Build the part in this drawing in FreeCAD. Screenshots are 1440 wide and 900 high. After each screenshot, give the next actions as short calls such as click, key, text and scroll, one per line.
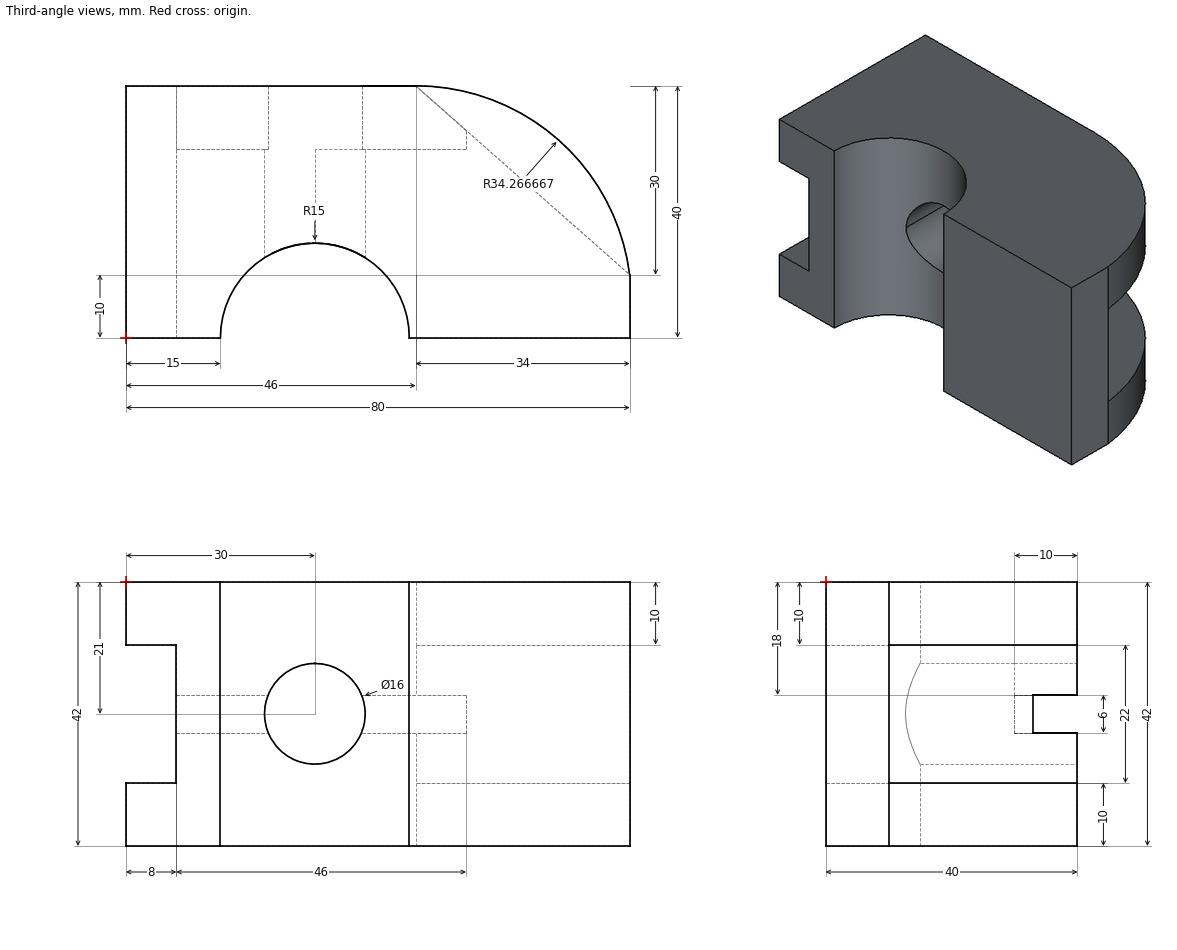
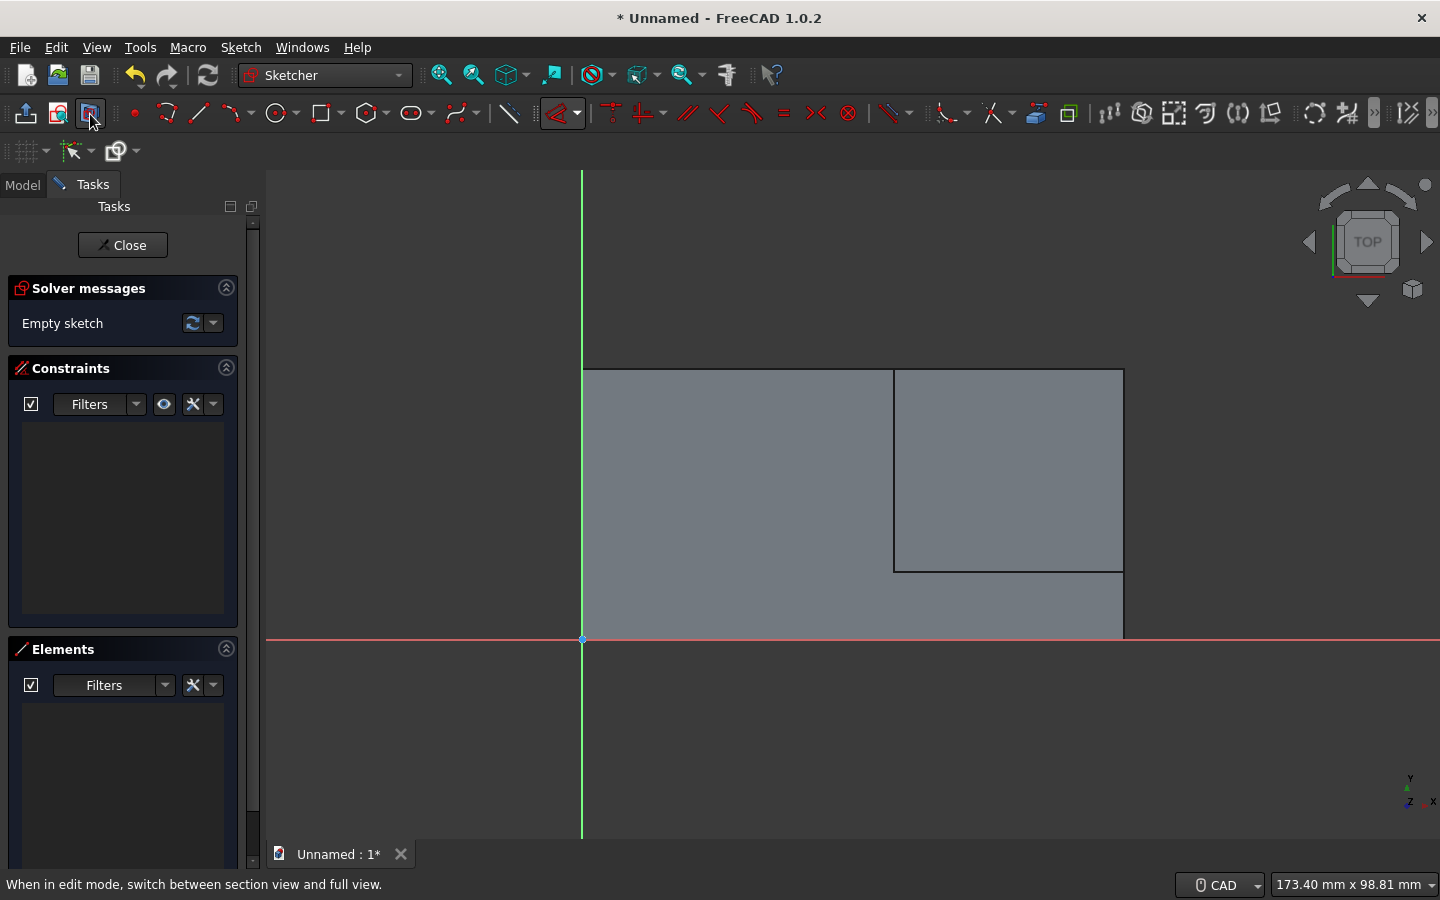
click(168, 114)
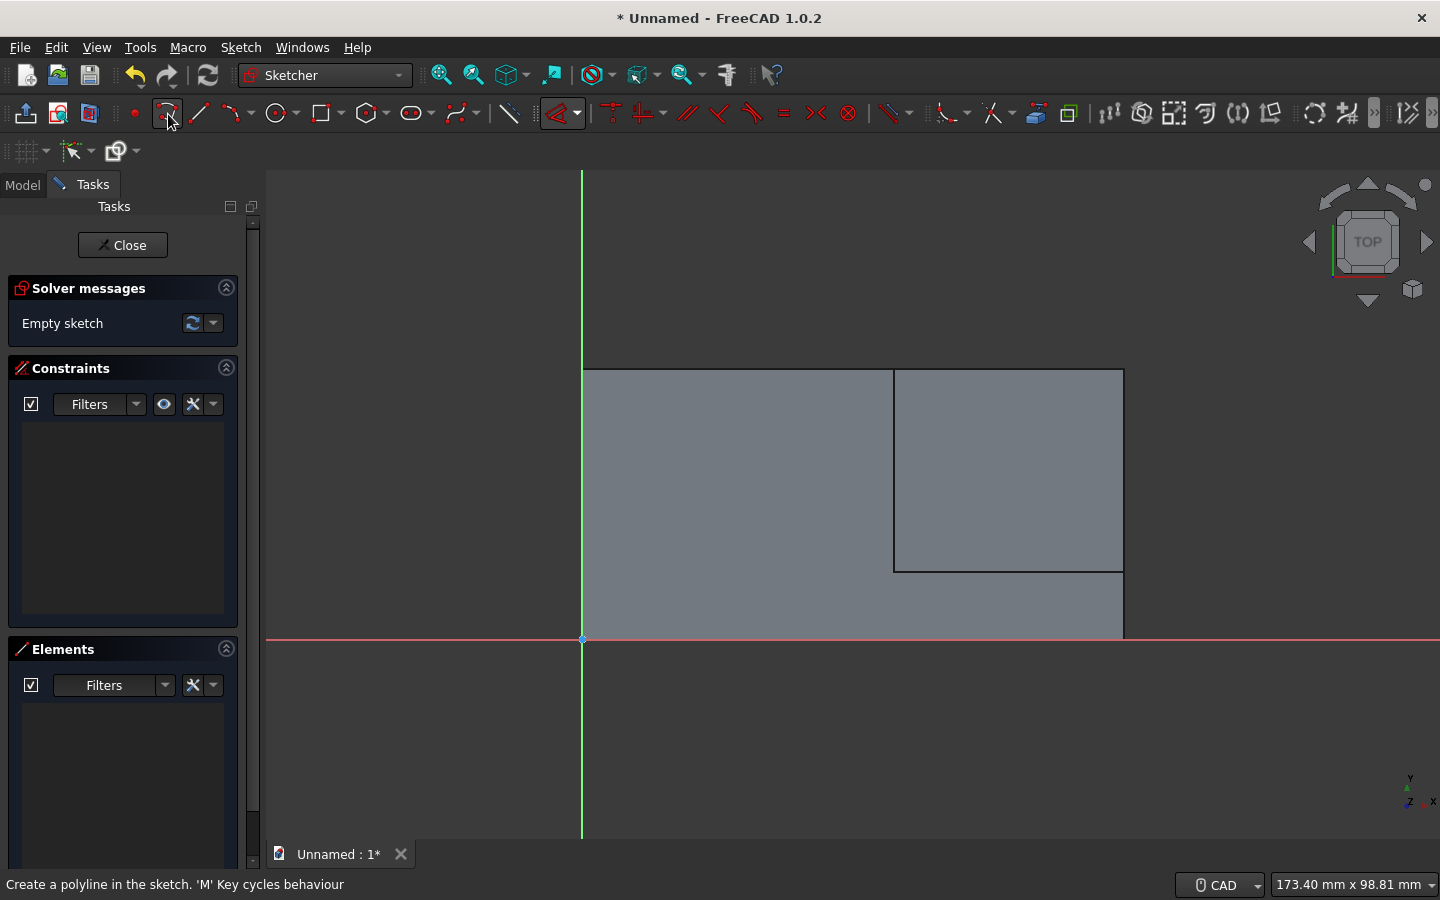
click(894, 369)
click(1124, 572)
click(1124, 369)
click(894, 370)
key(Escape)
key(Escape)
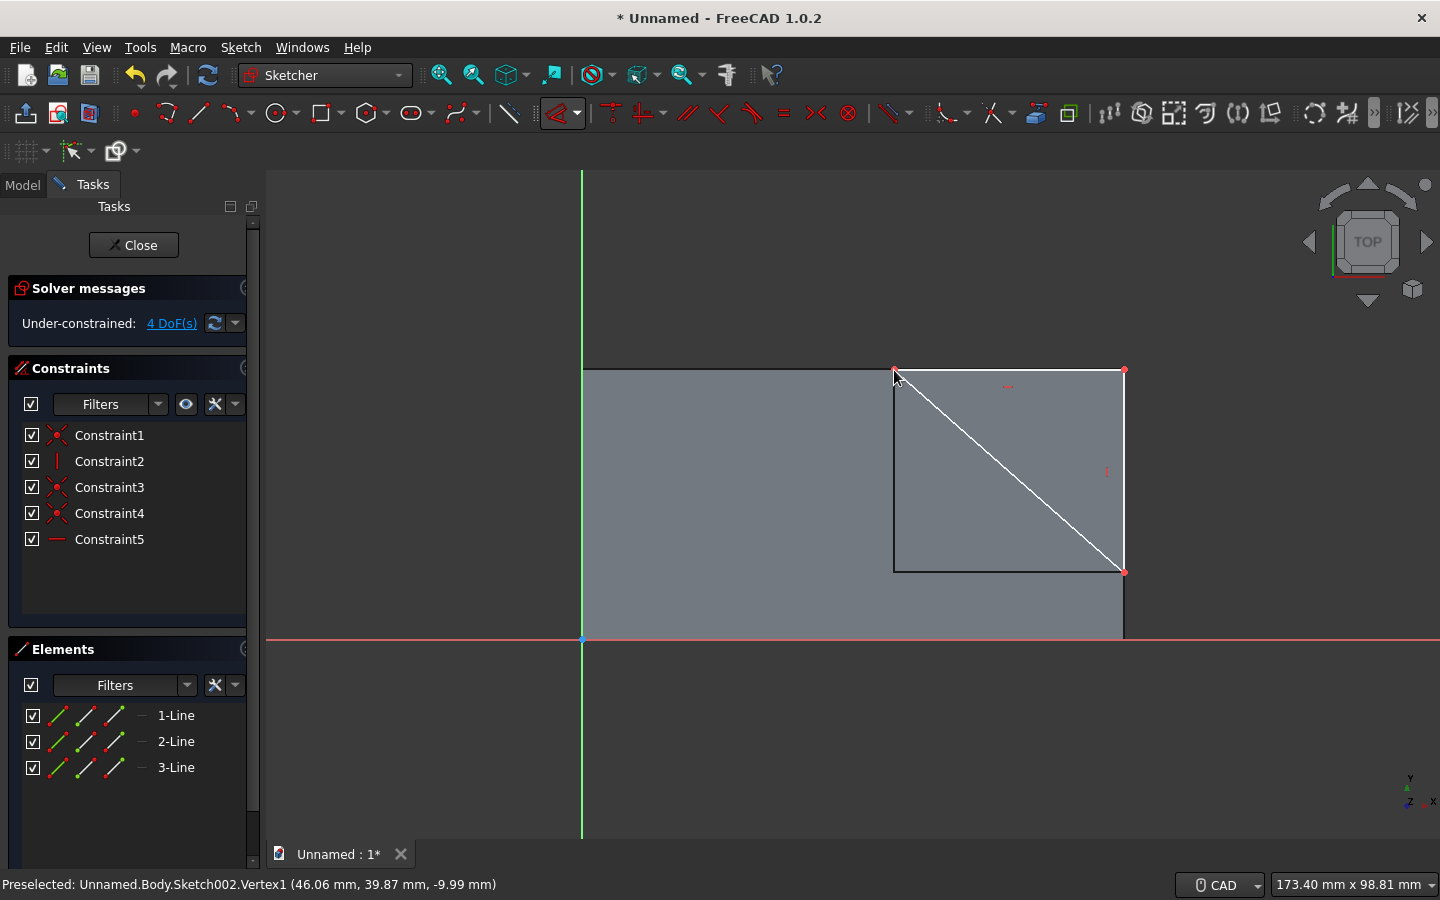
click(1124, 512)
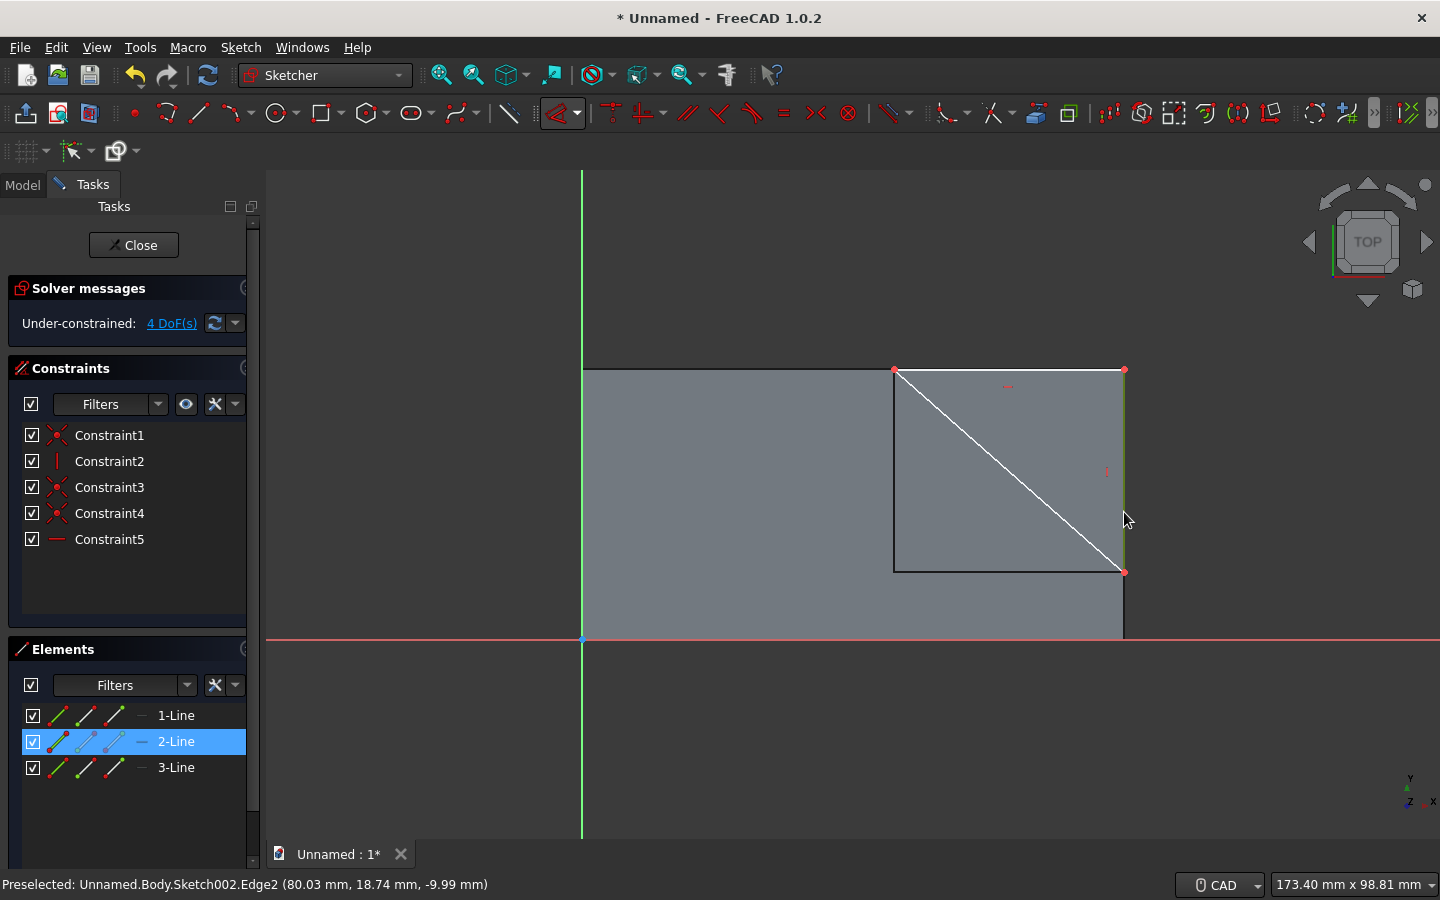
key(i)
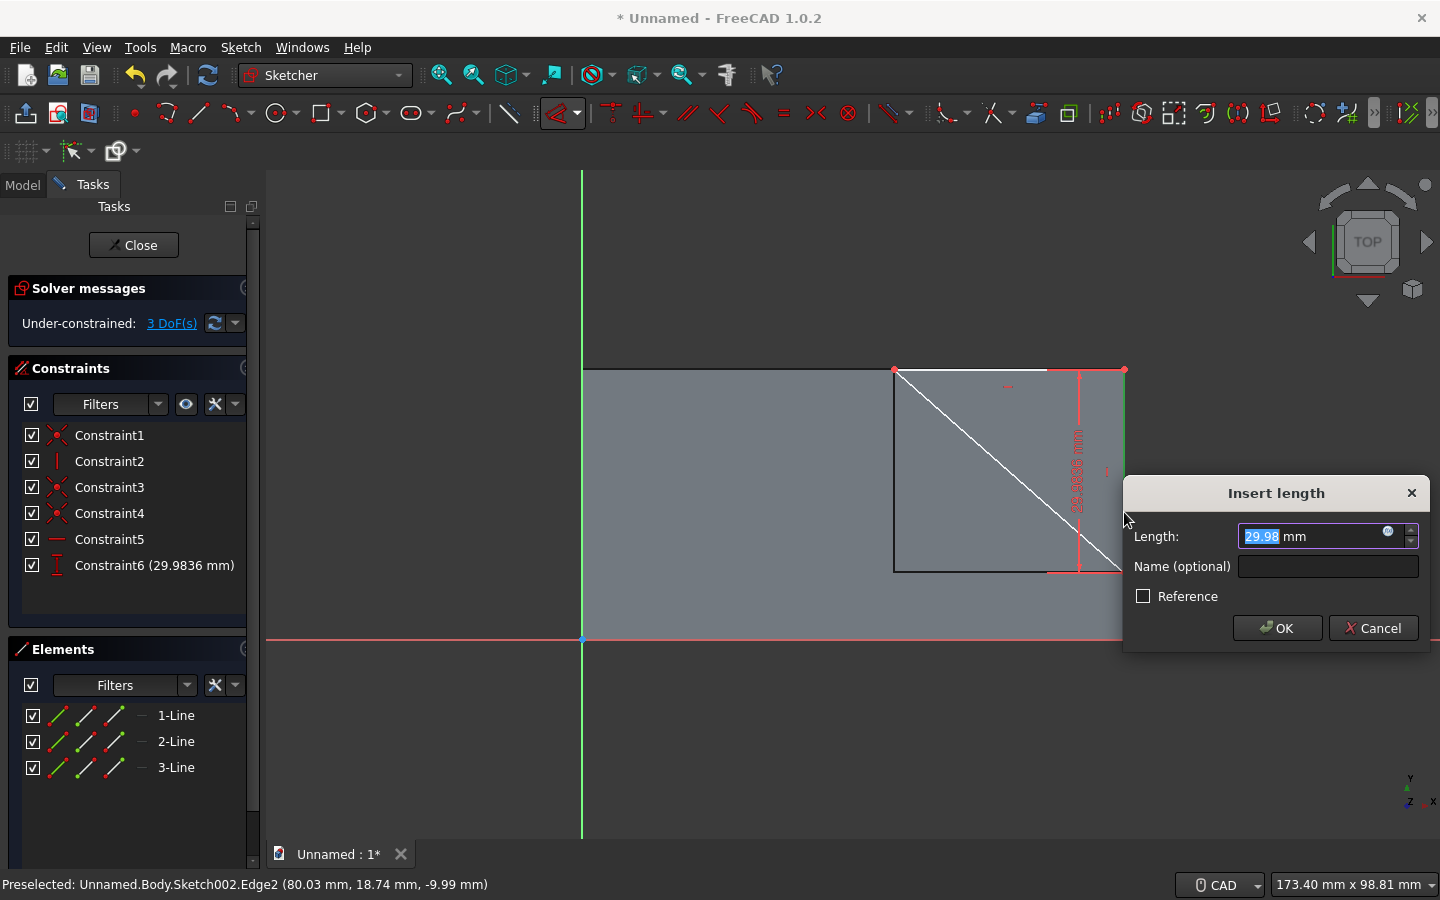
text(30)
key(Return)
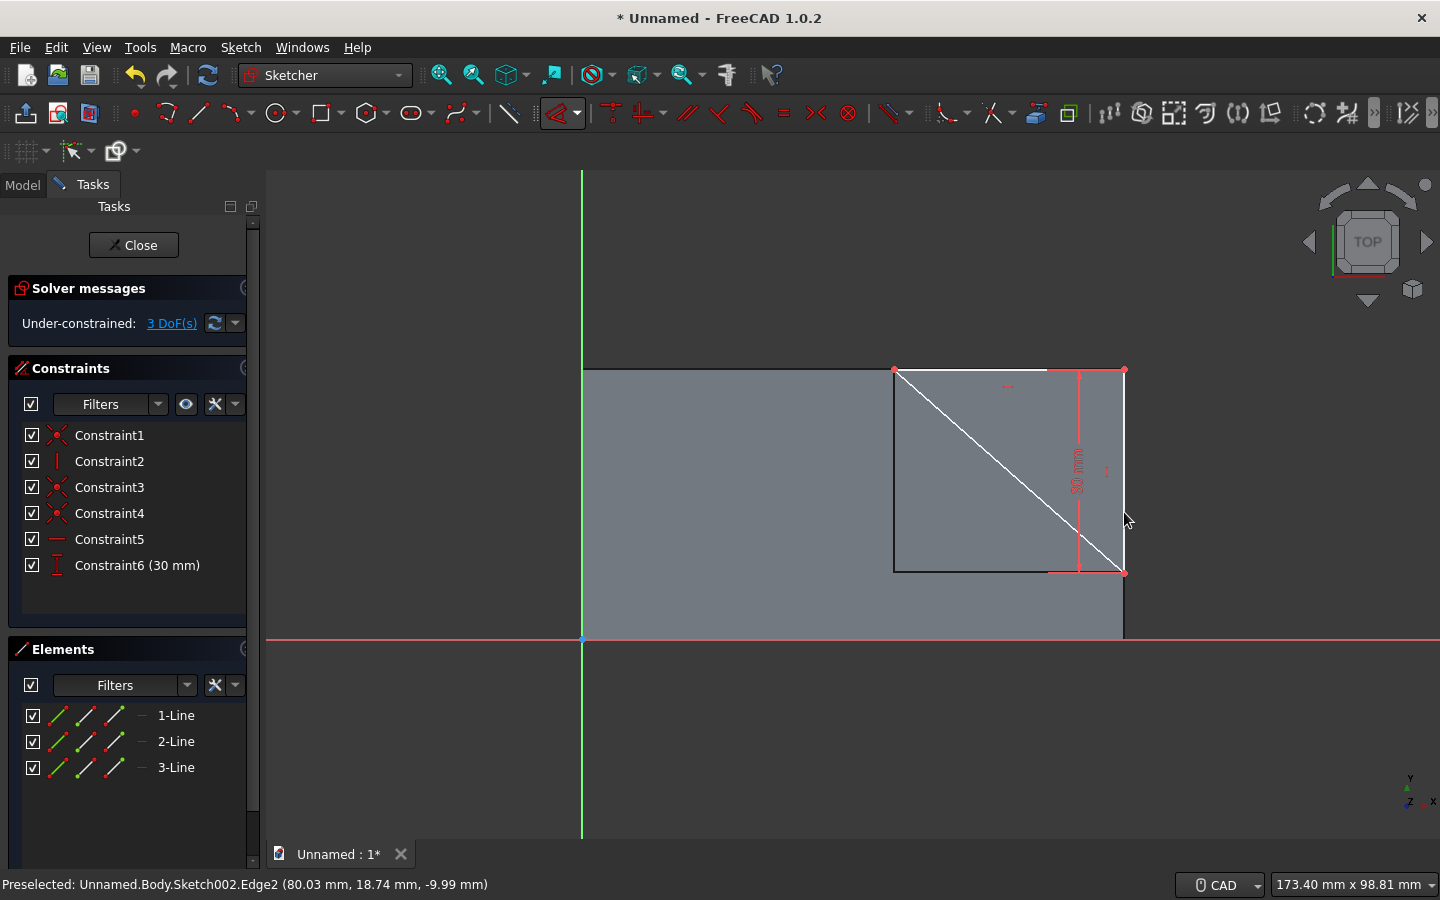
click(1055, 370)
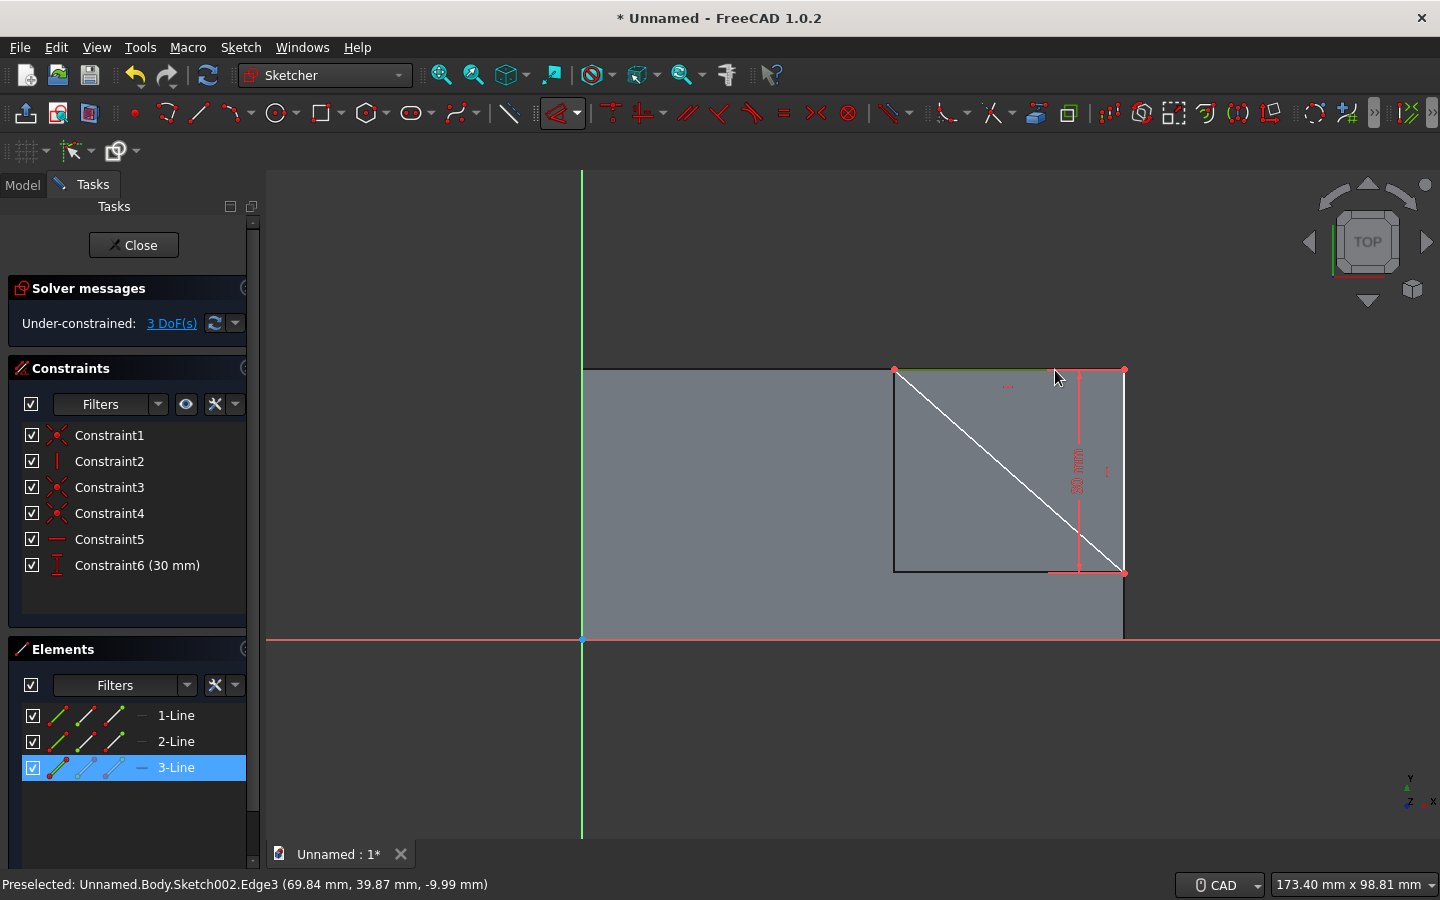
key(l)